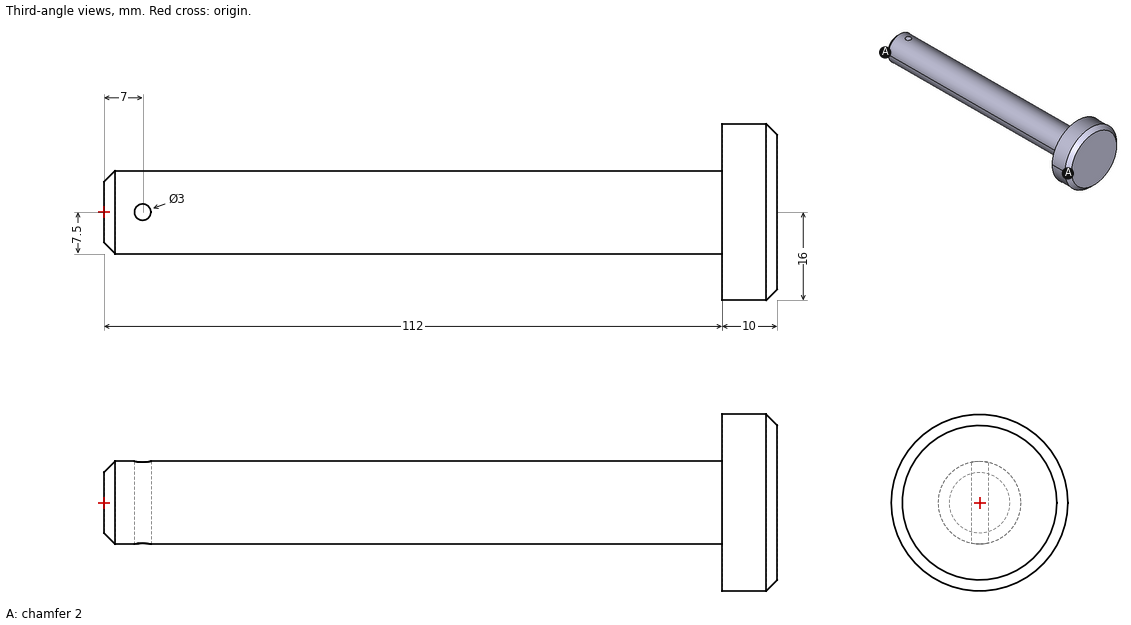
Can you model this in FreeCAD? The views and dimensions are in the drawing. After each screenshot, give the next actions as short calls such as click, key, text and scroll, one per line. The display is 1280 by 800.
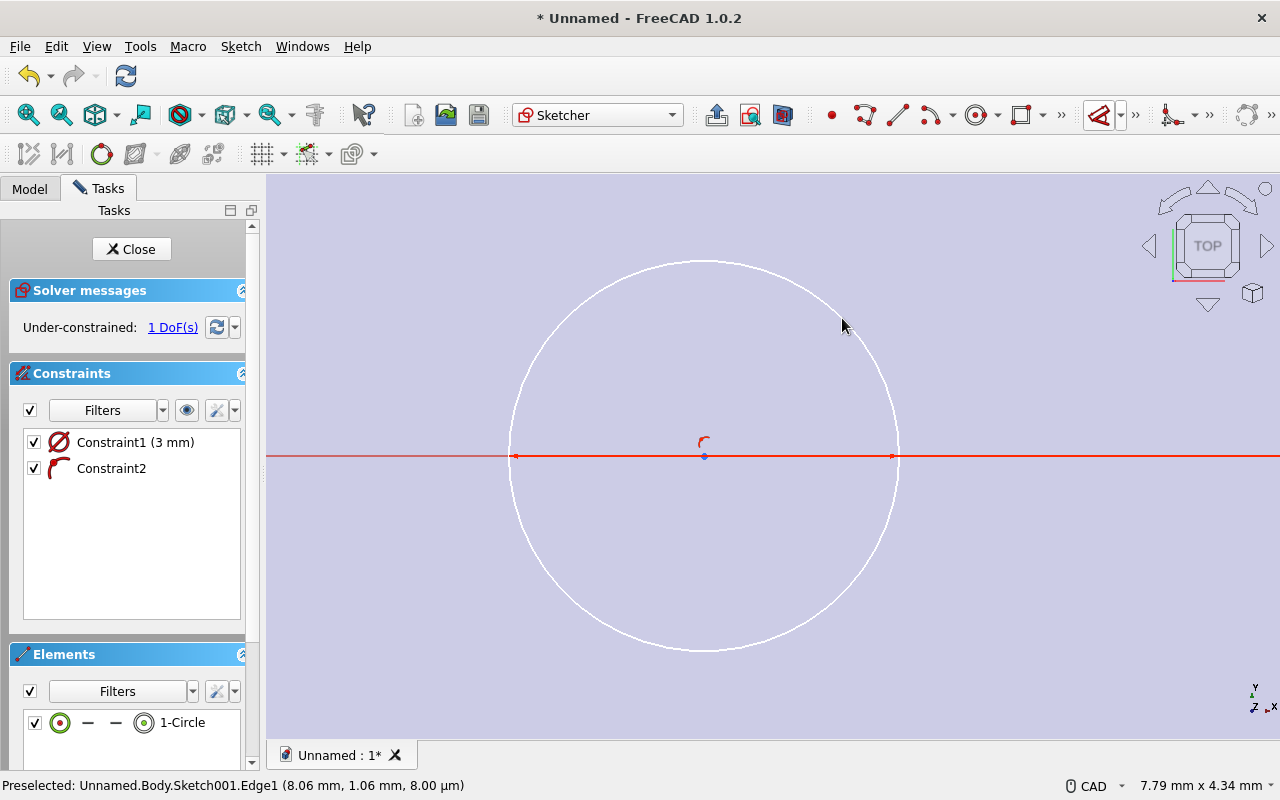
click(704, 456)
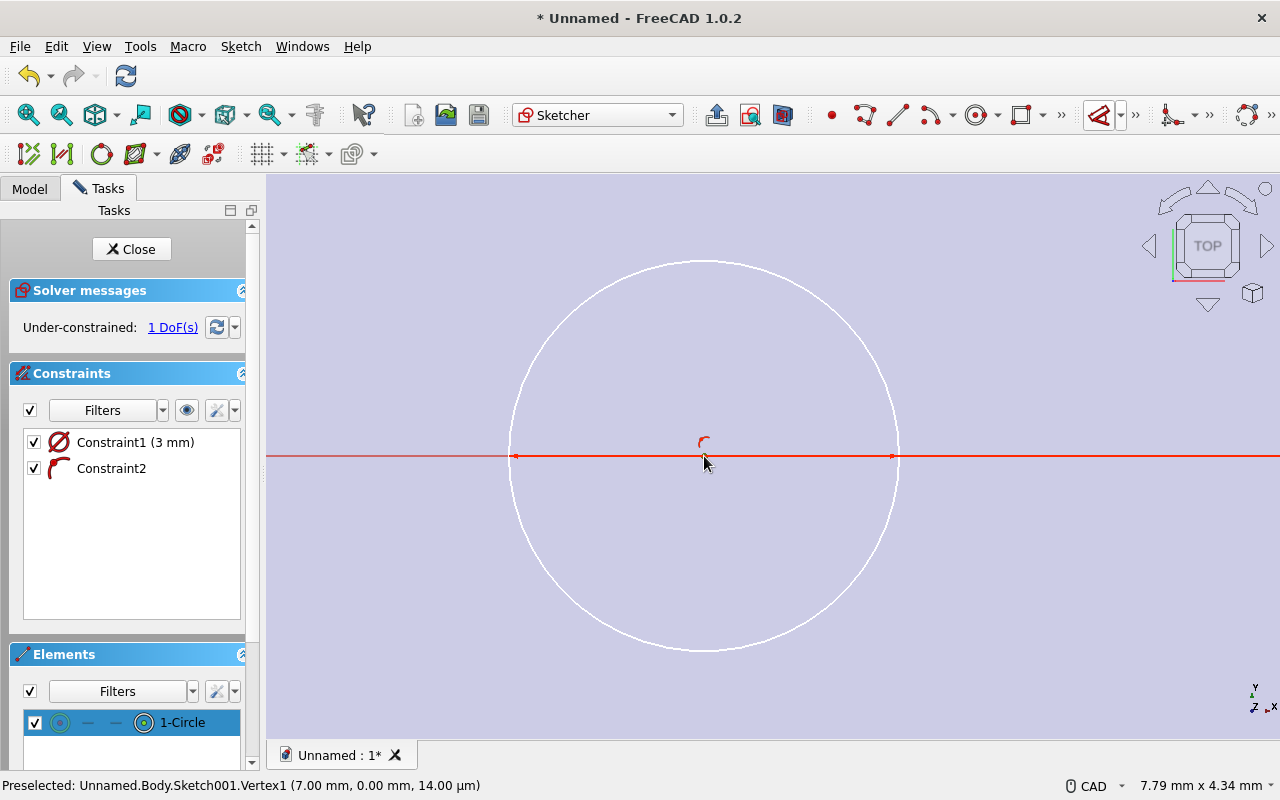
key(l)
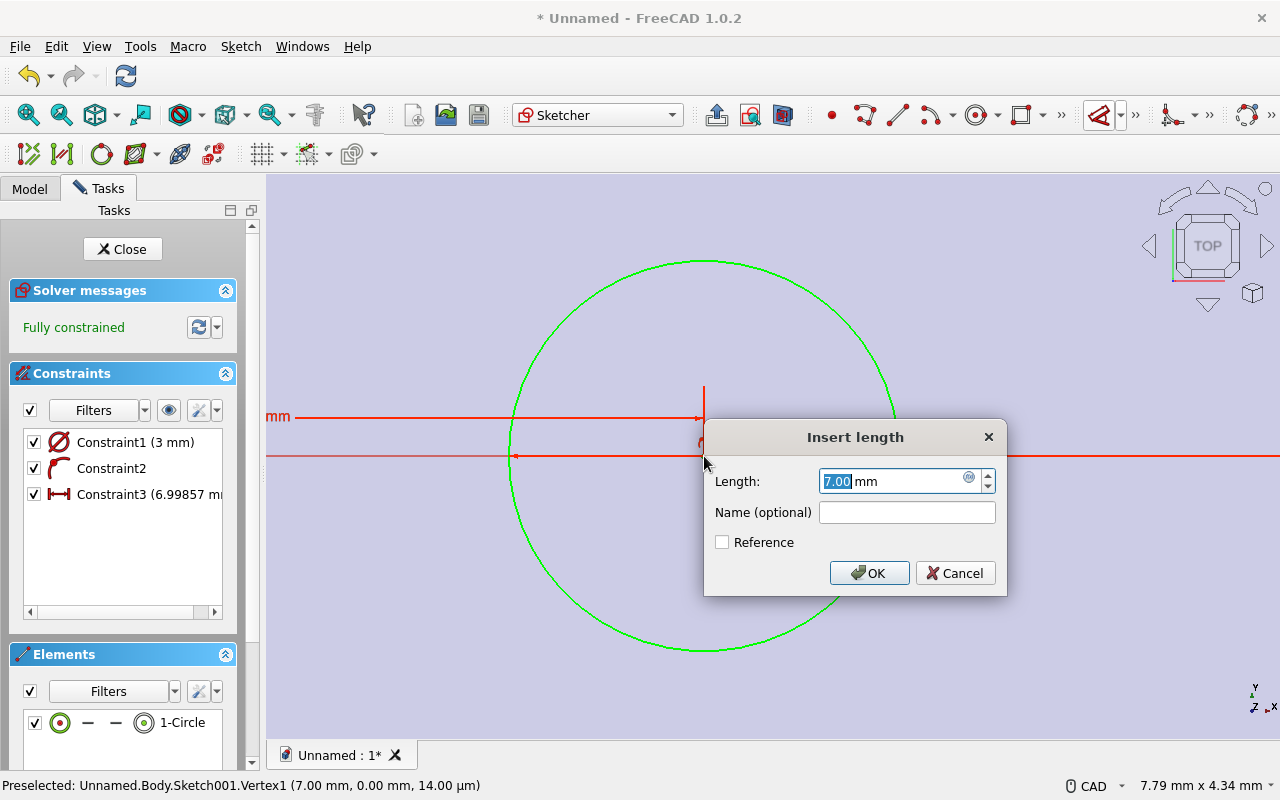
text(7)
key(Return)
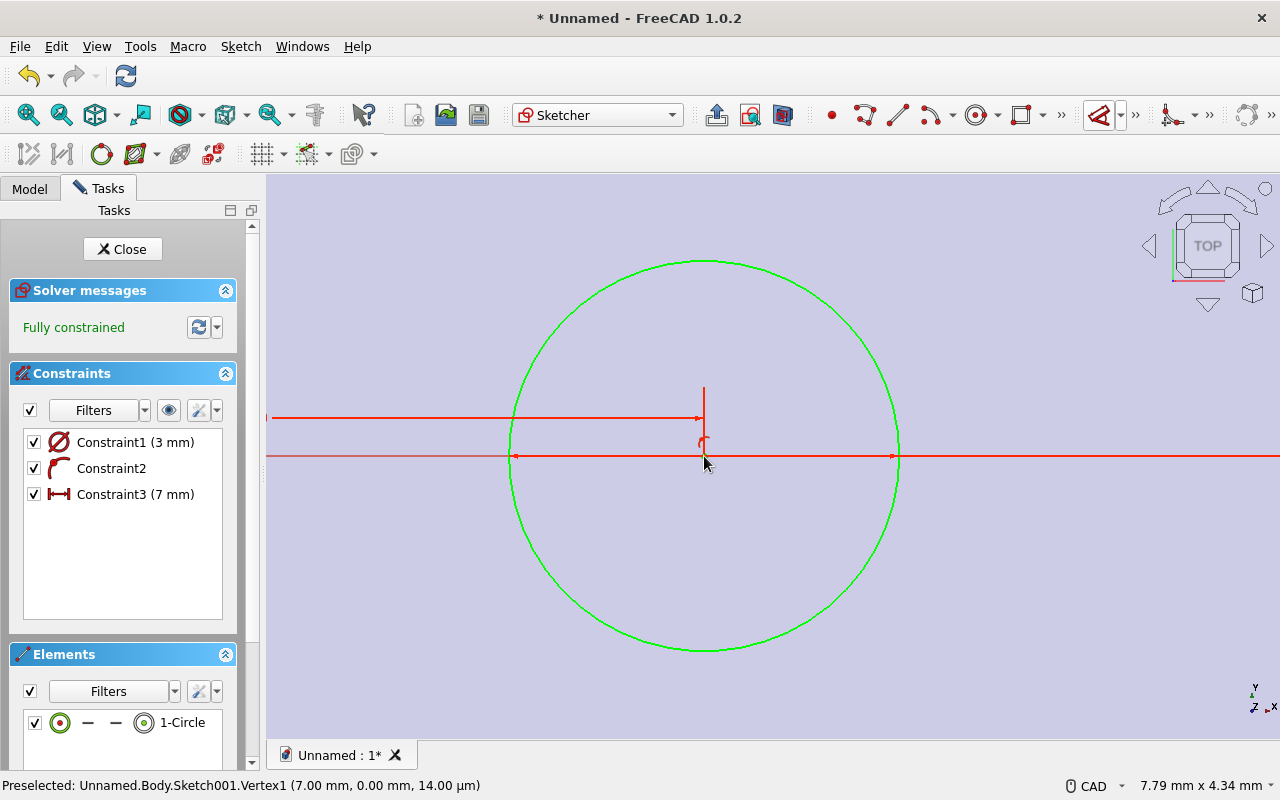
click(123, 249)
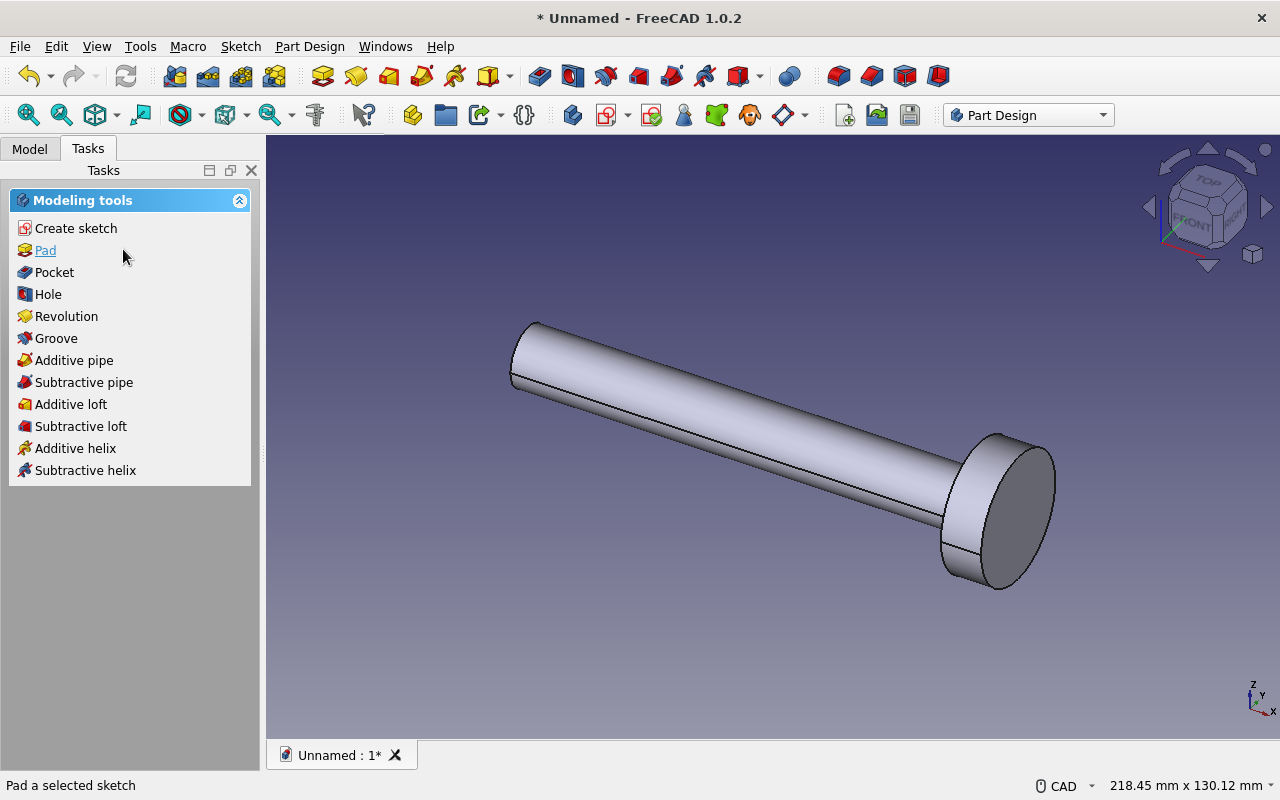
click(540, 76)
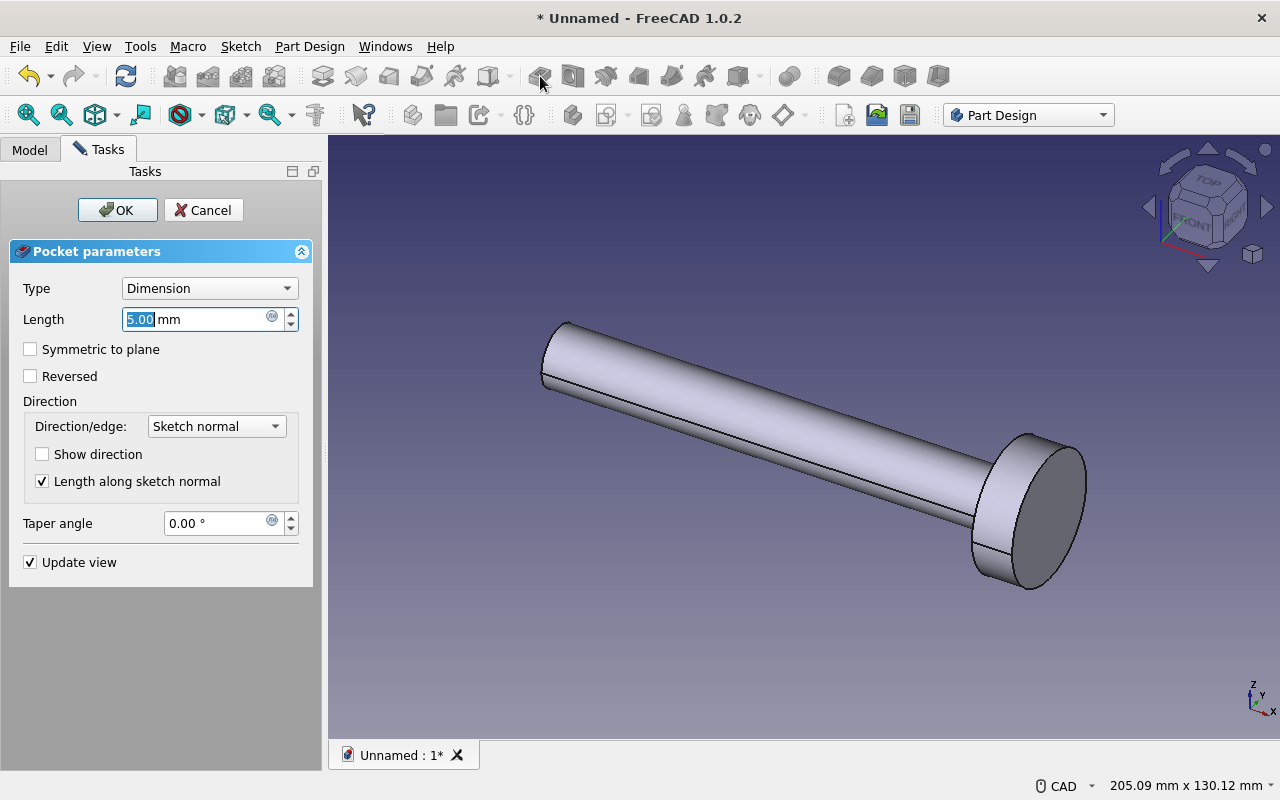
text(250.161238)
key(Tab)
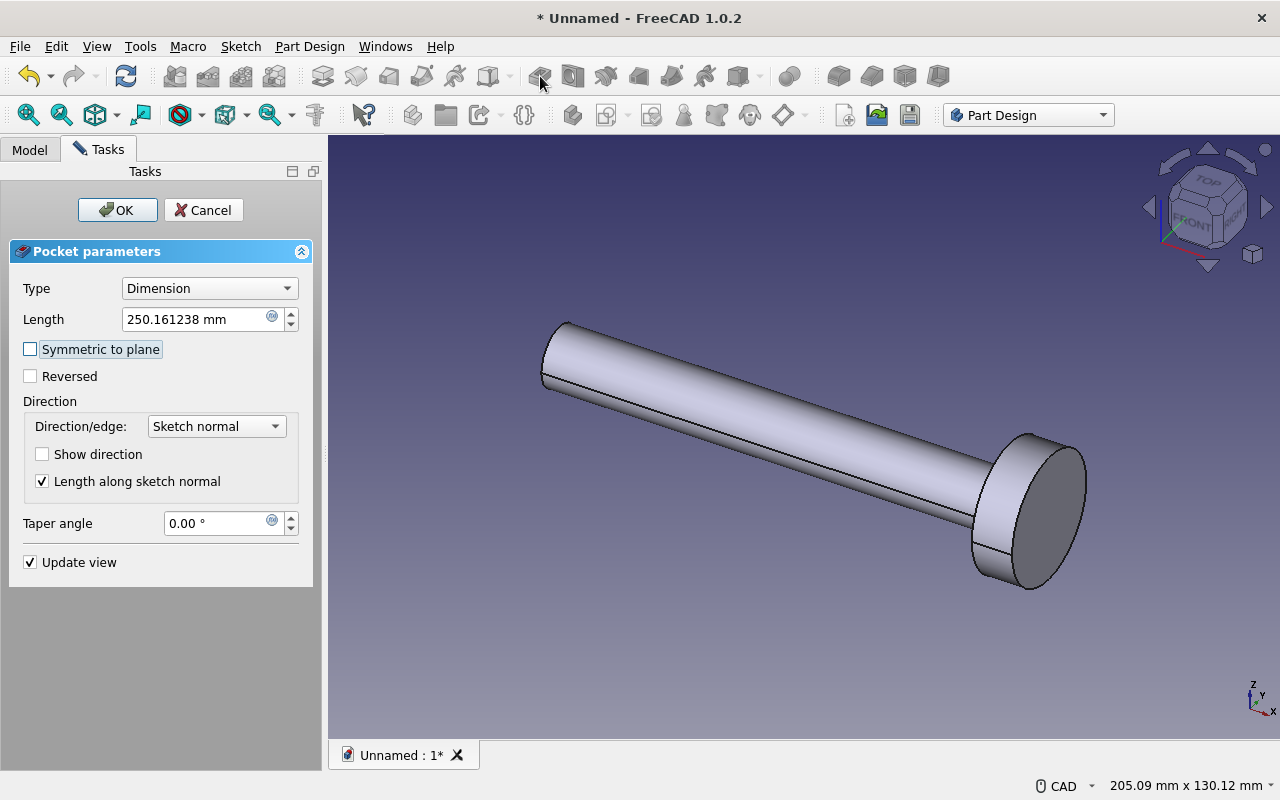
click(31, 349)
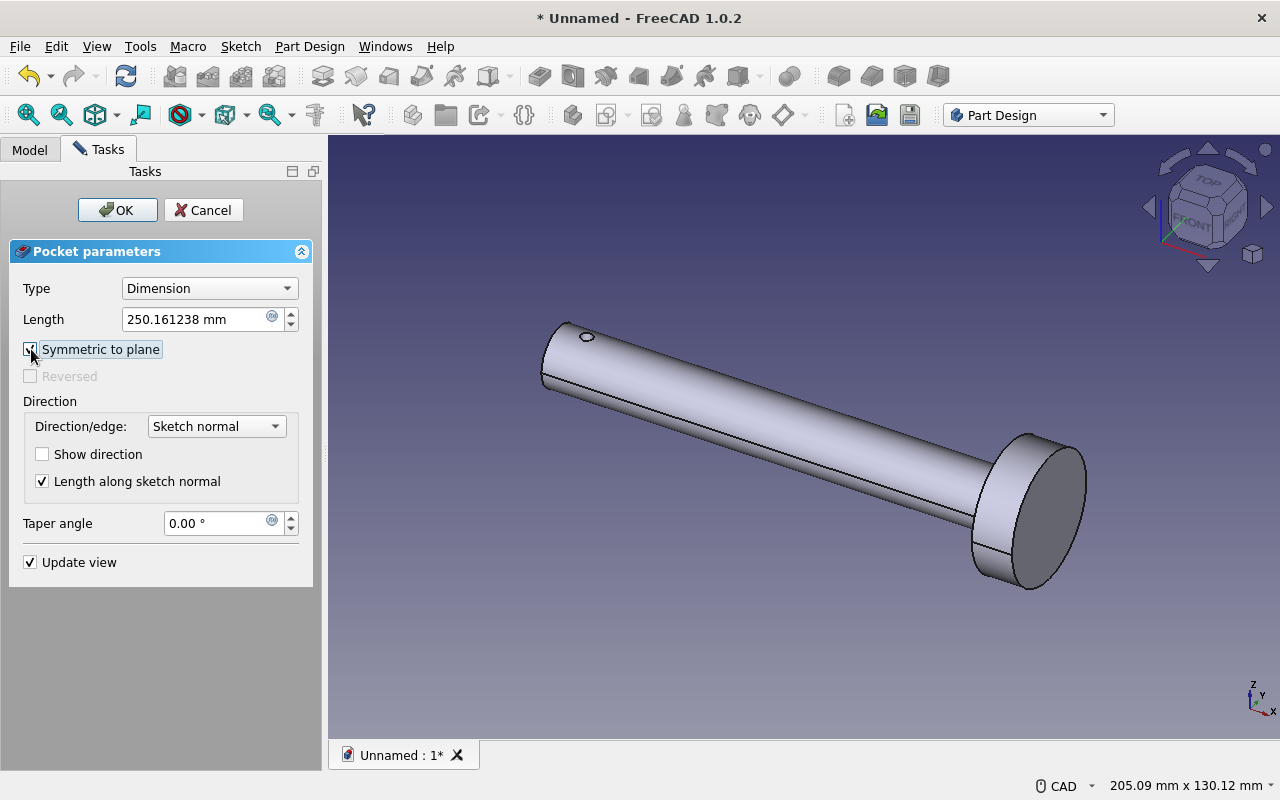
click(118, 210)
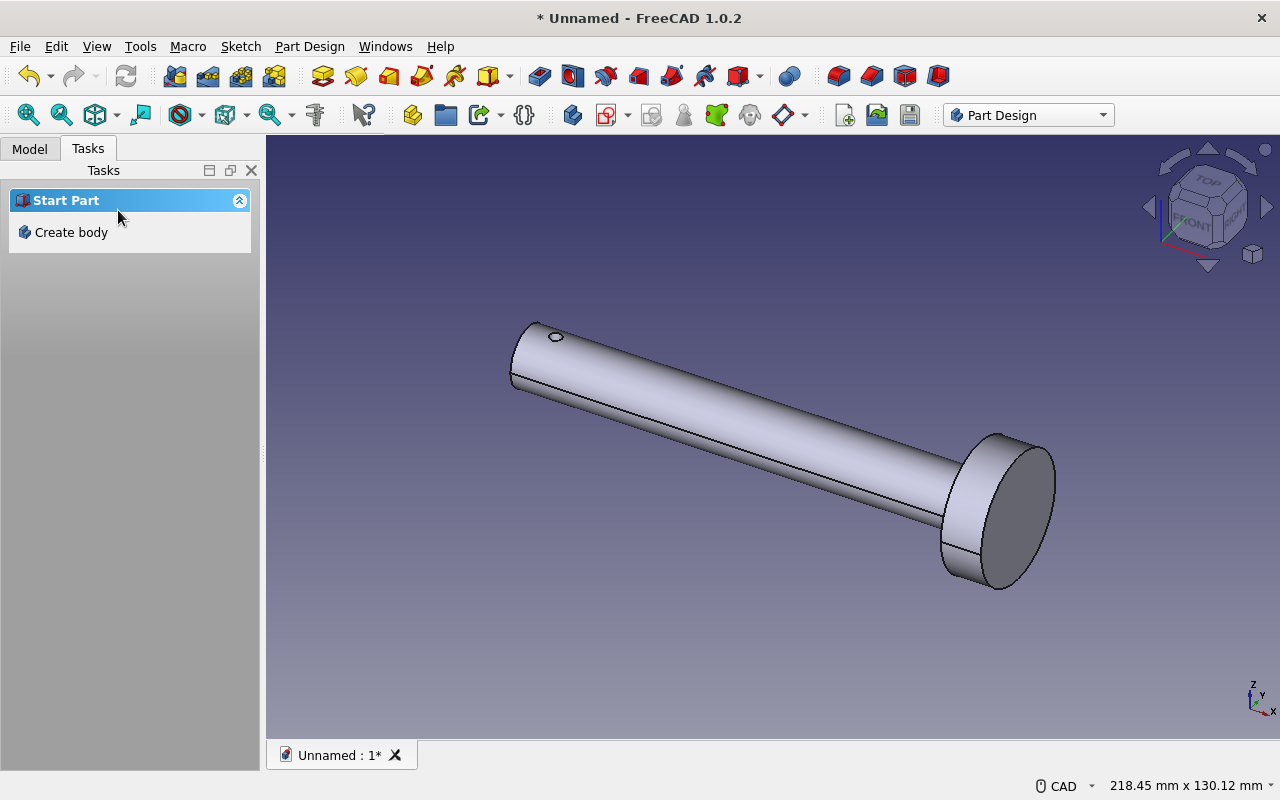
click(1030, 448)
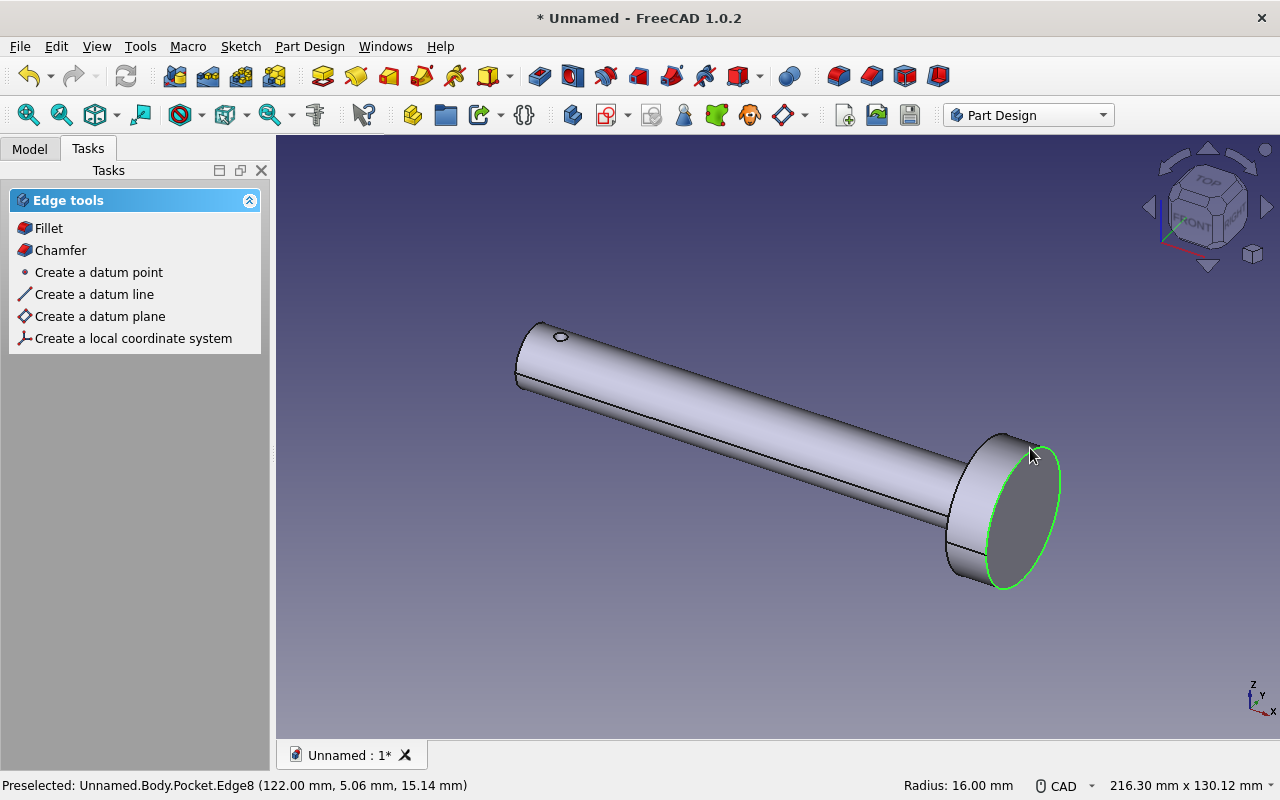
click(527, 333, ctrl)